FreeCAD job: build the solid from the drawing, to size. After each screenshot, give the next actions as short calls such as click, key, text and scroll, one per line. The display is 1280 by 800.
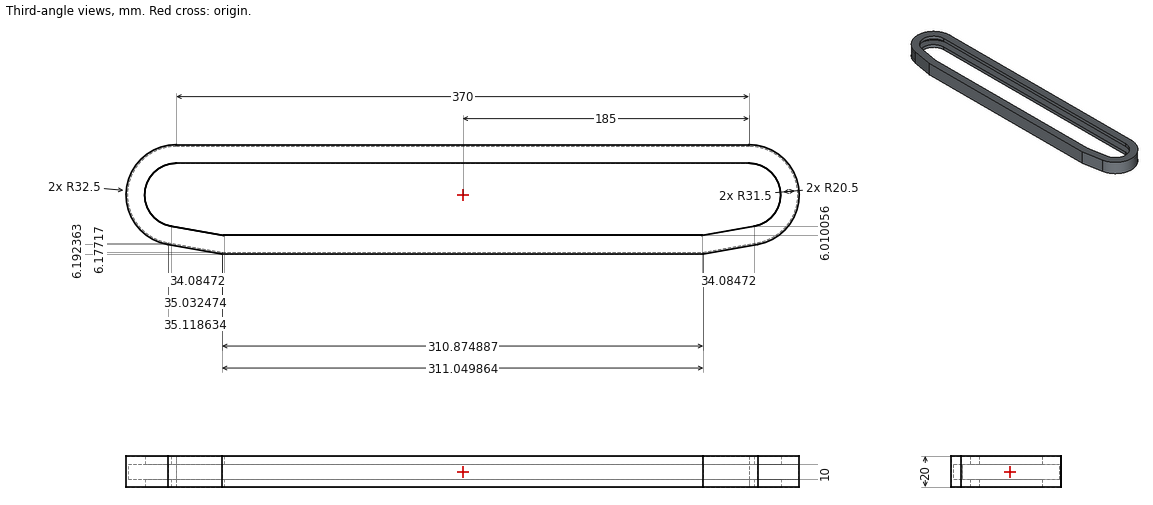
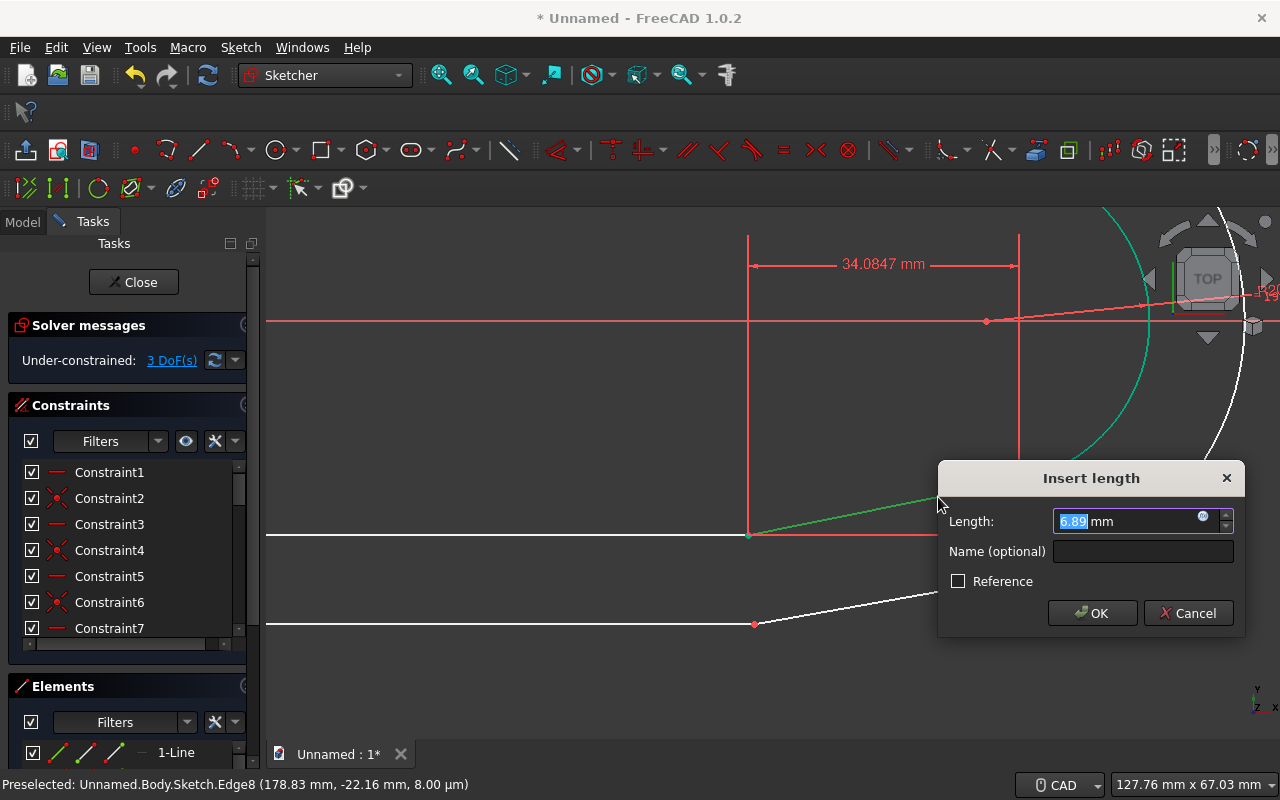
text(6.010056)
key(Return)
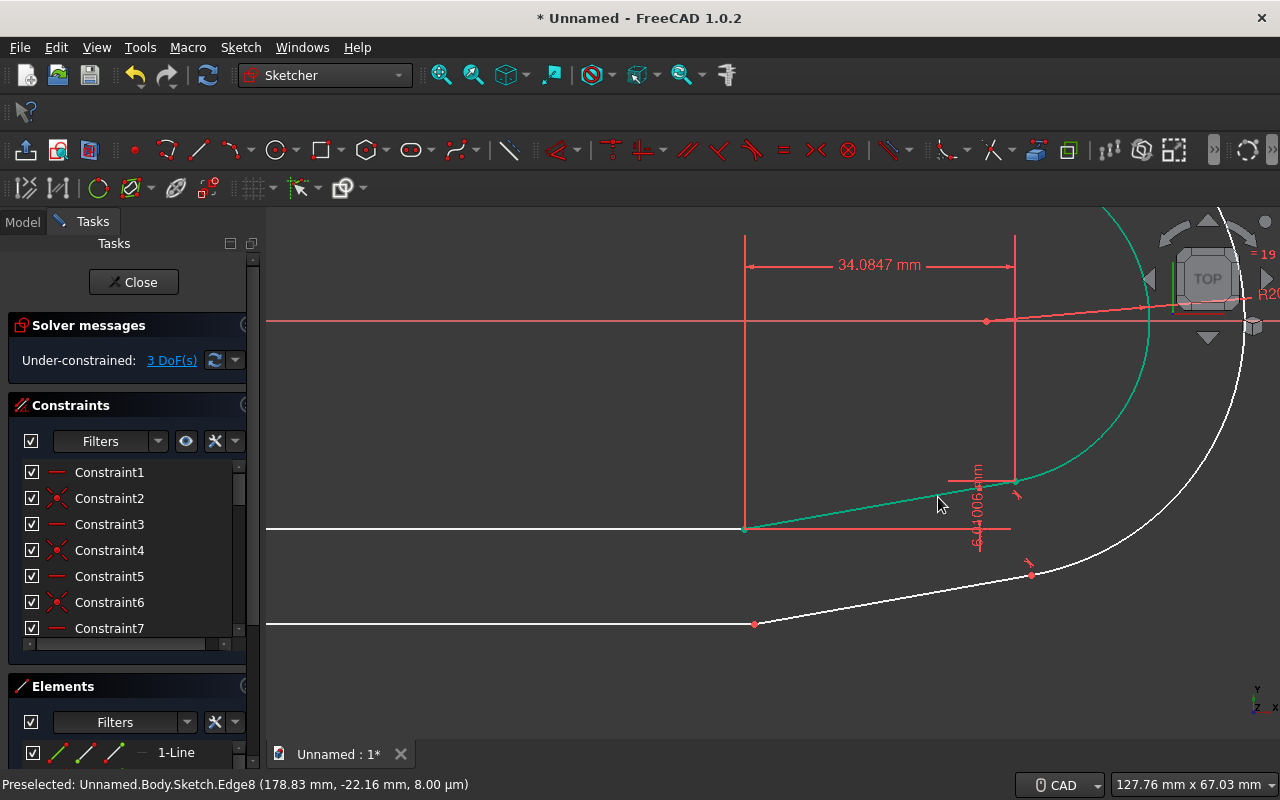
scroll(939, 499, down, 9)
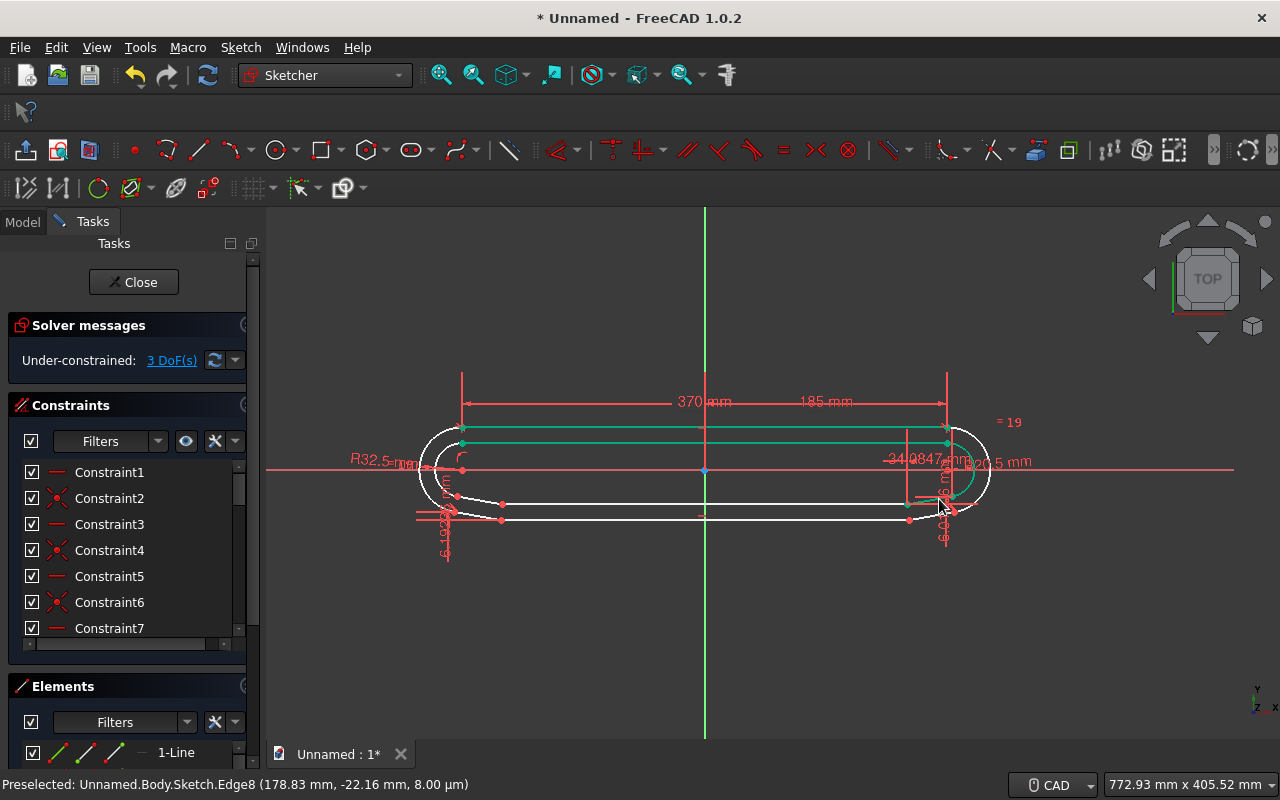
click(489, 502)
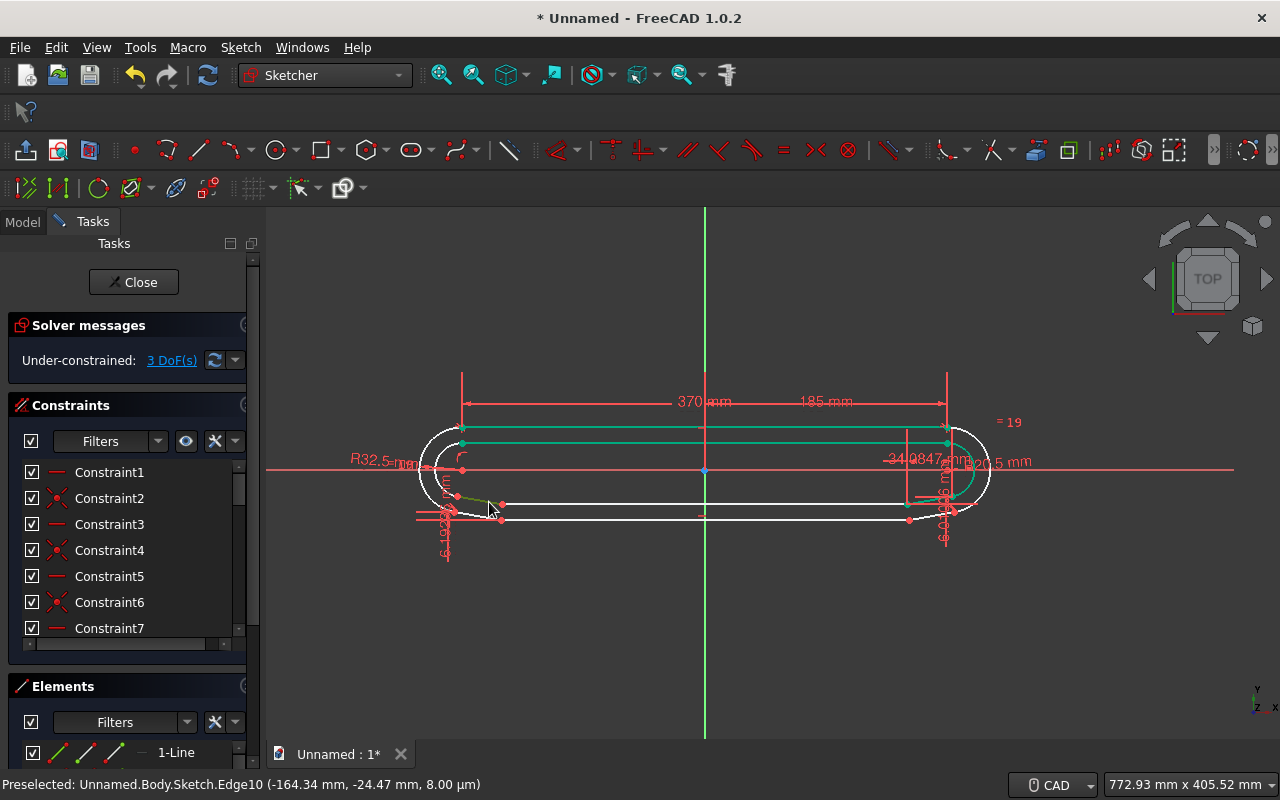
key(l)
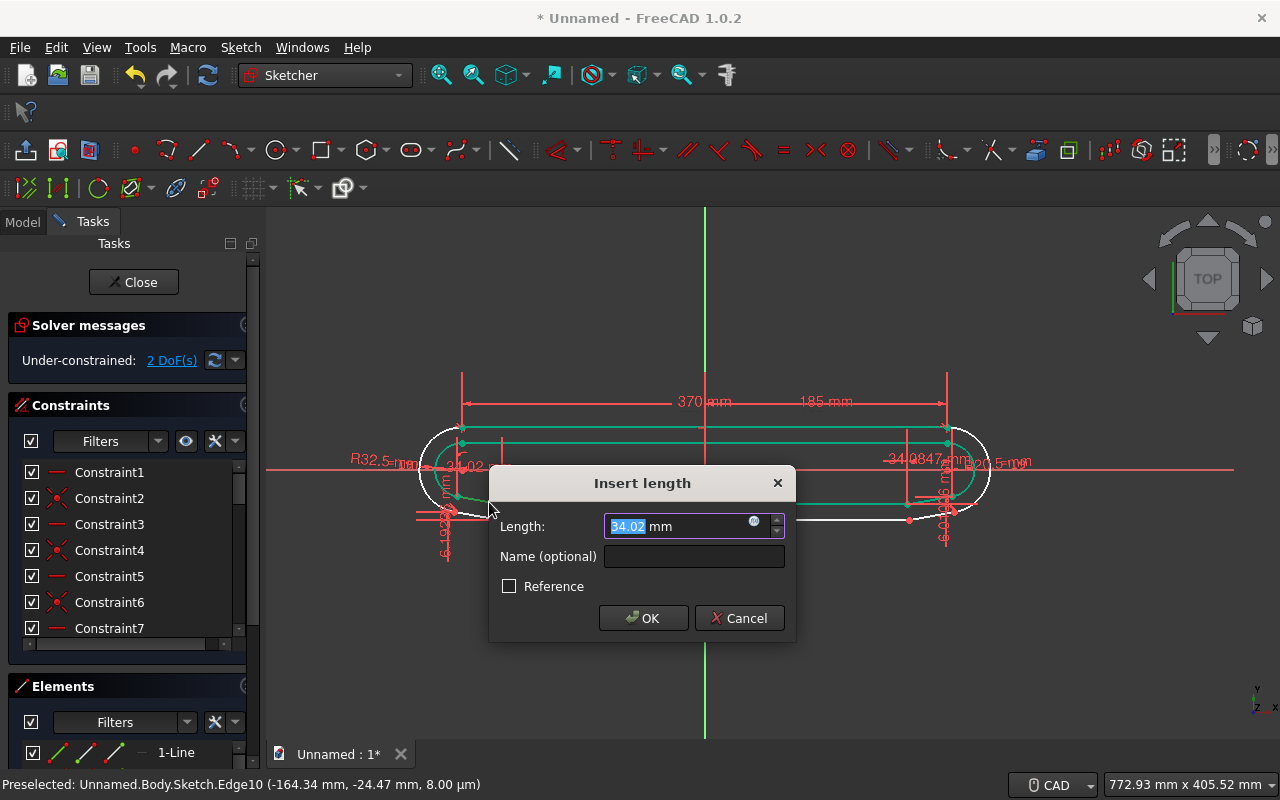
text(34.08472)
key(Return)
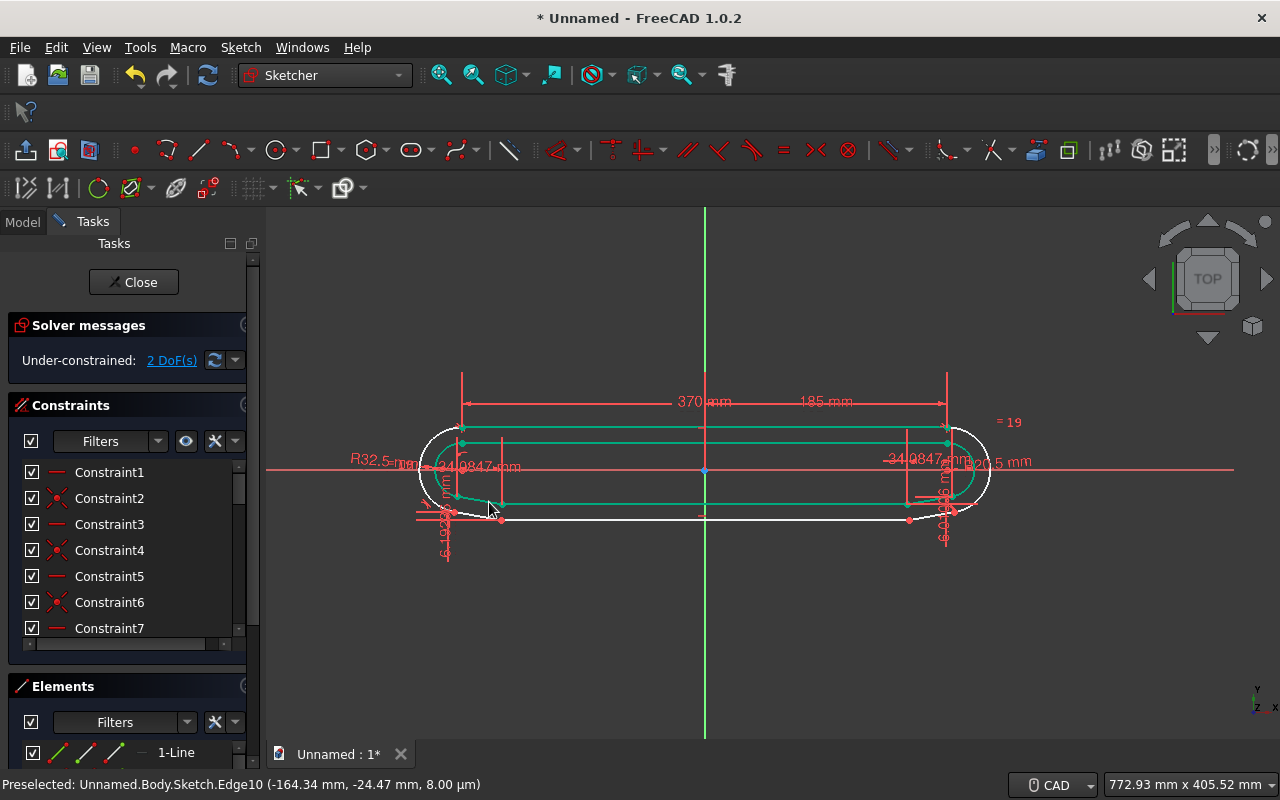
click(623, 520)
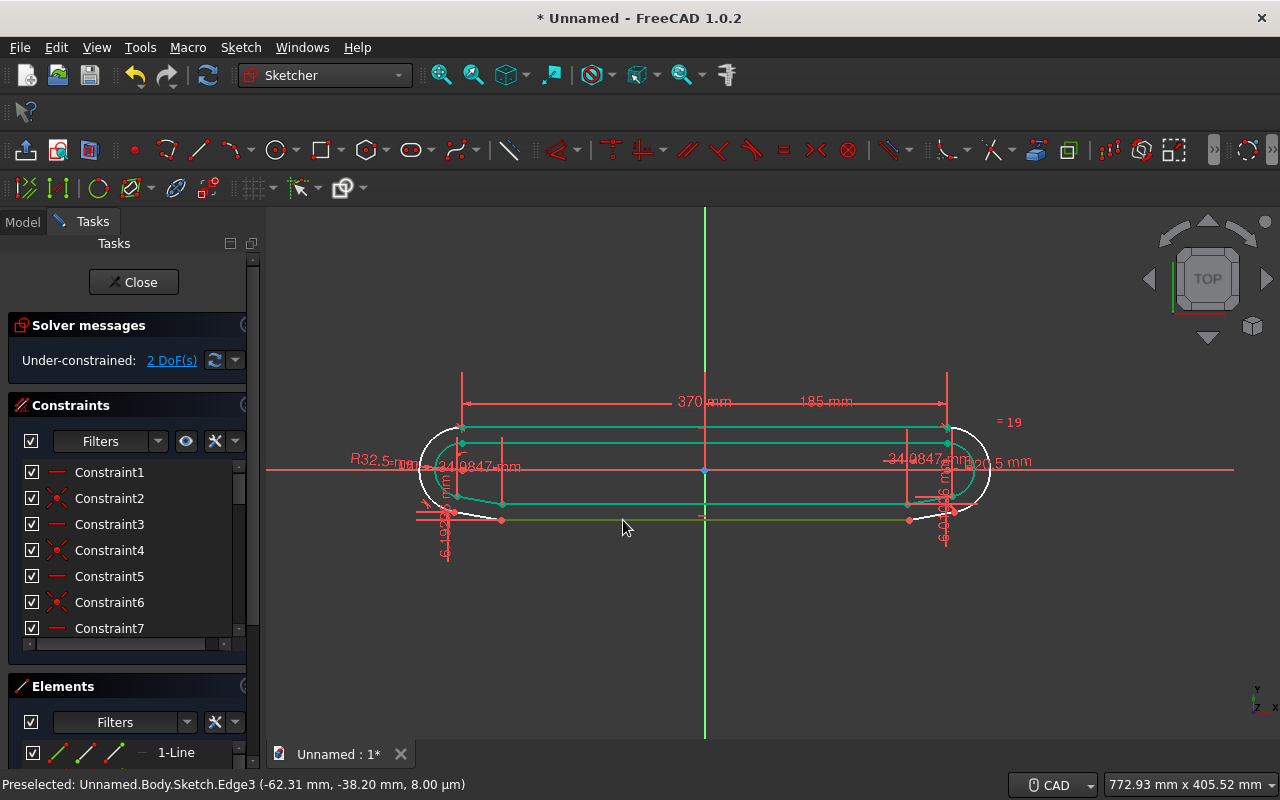
click(580, 150)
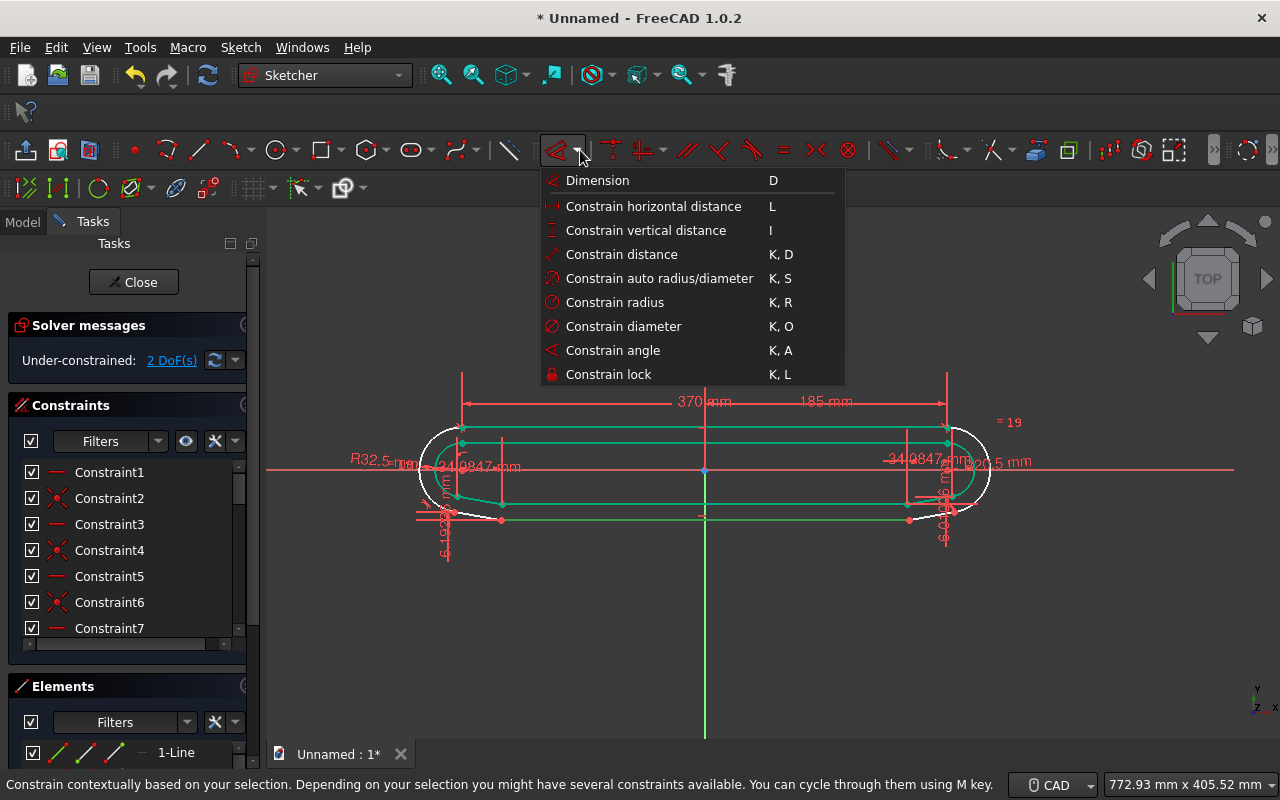
click(693, 206)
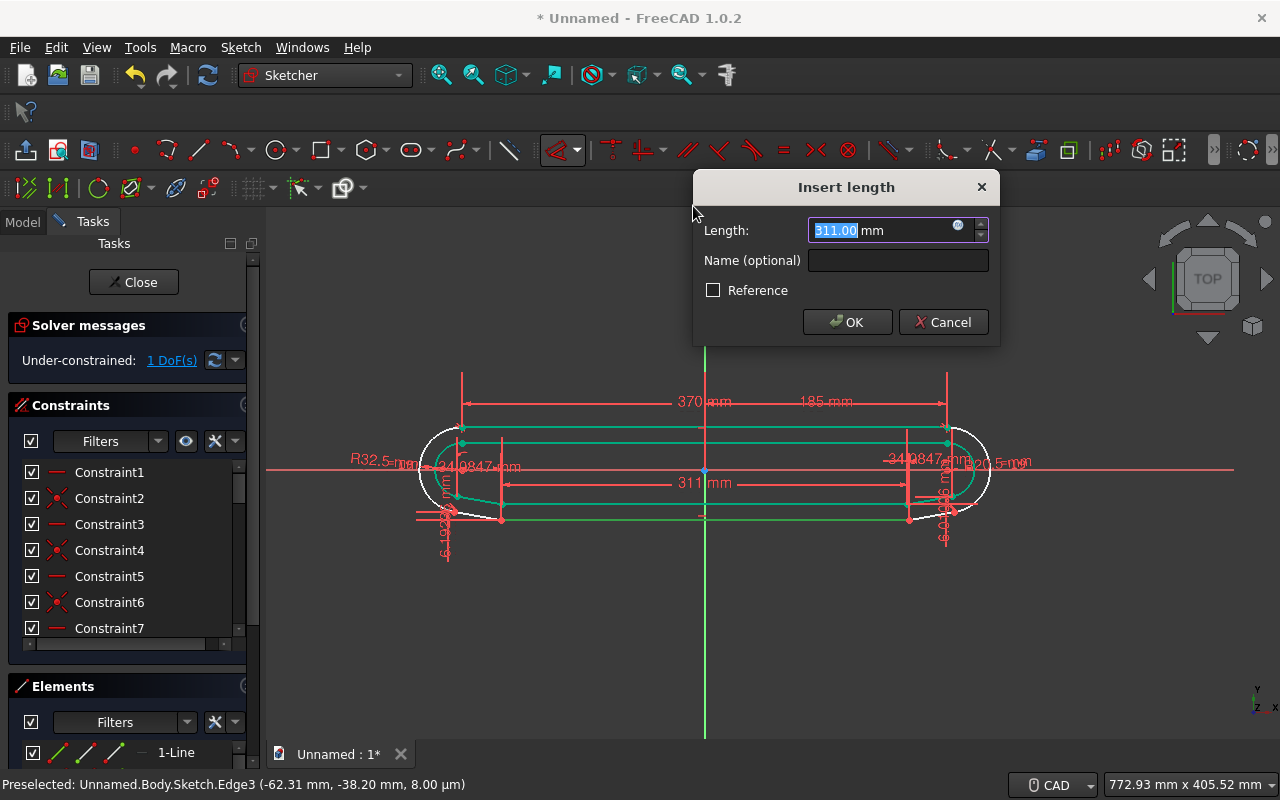
text(311.049864)
key(Return)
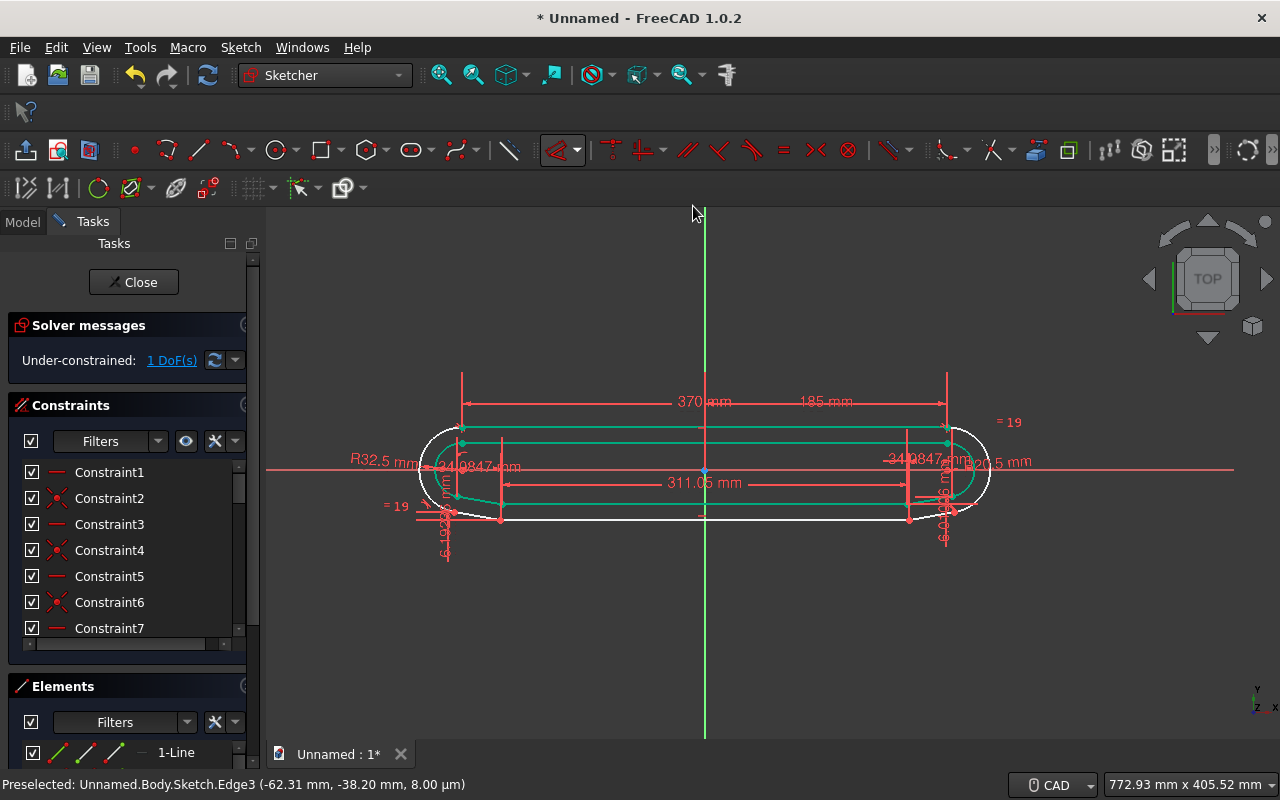
click(469, 515)